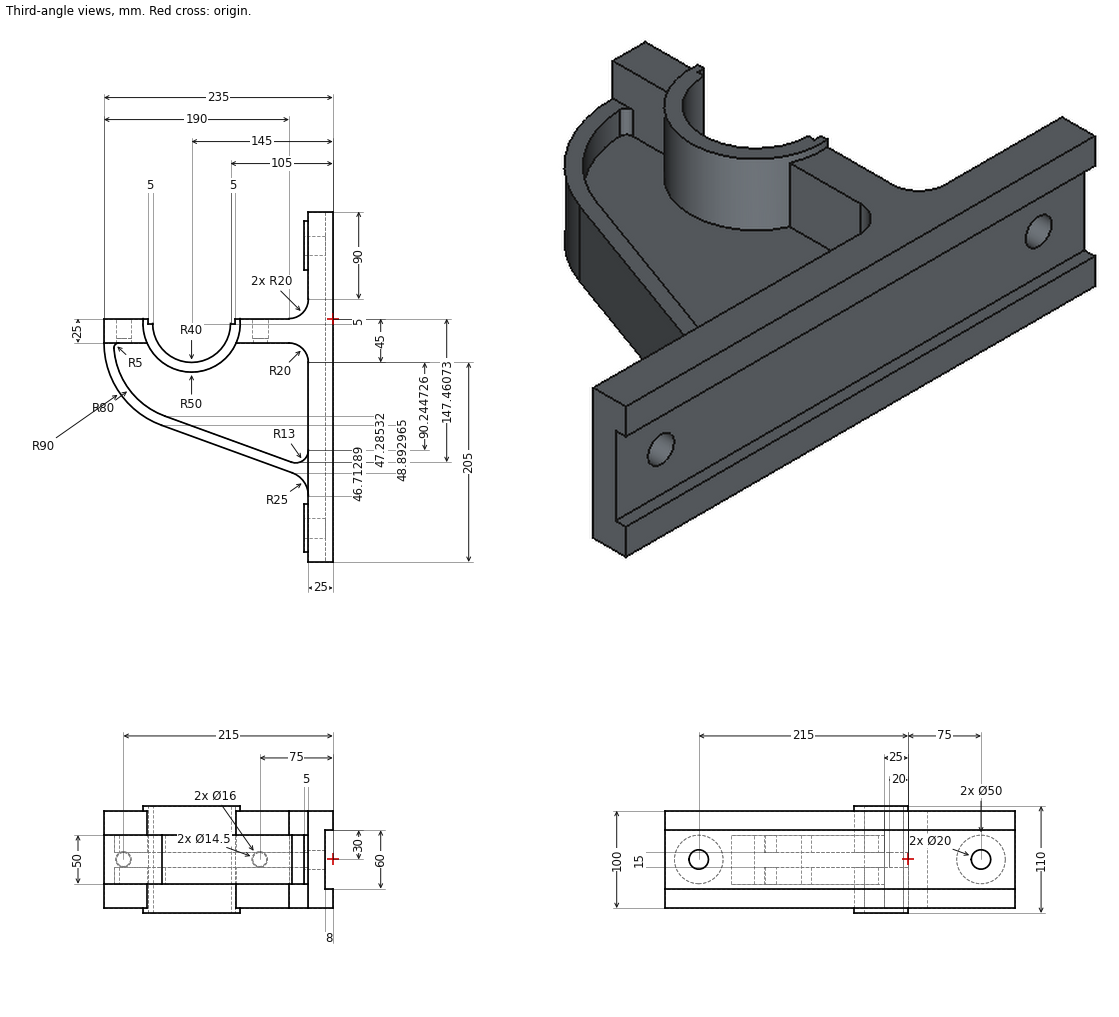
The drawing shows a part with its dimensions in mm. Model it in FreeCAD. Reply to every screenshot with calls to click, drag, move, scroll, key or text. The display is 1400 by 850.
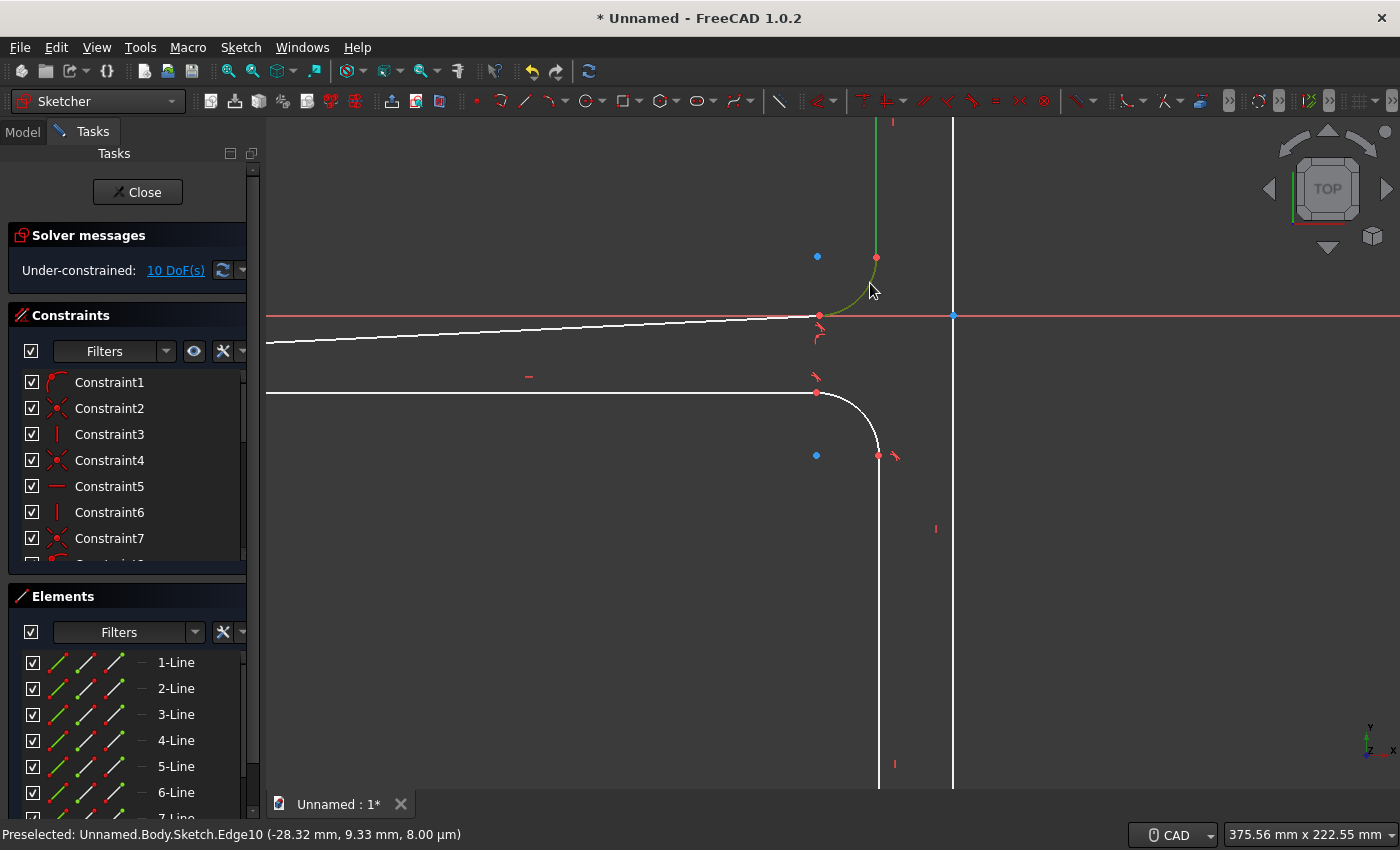
click(972, 102)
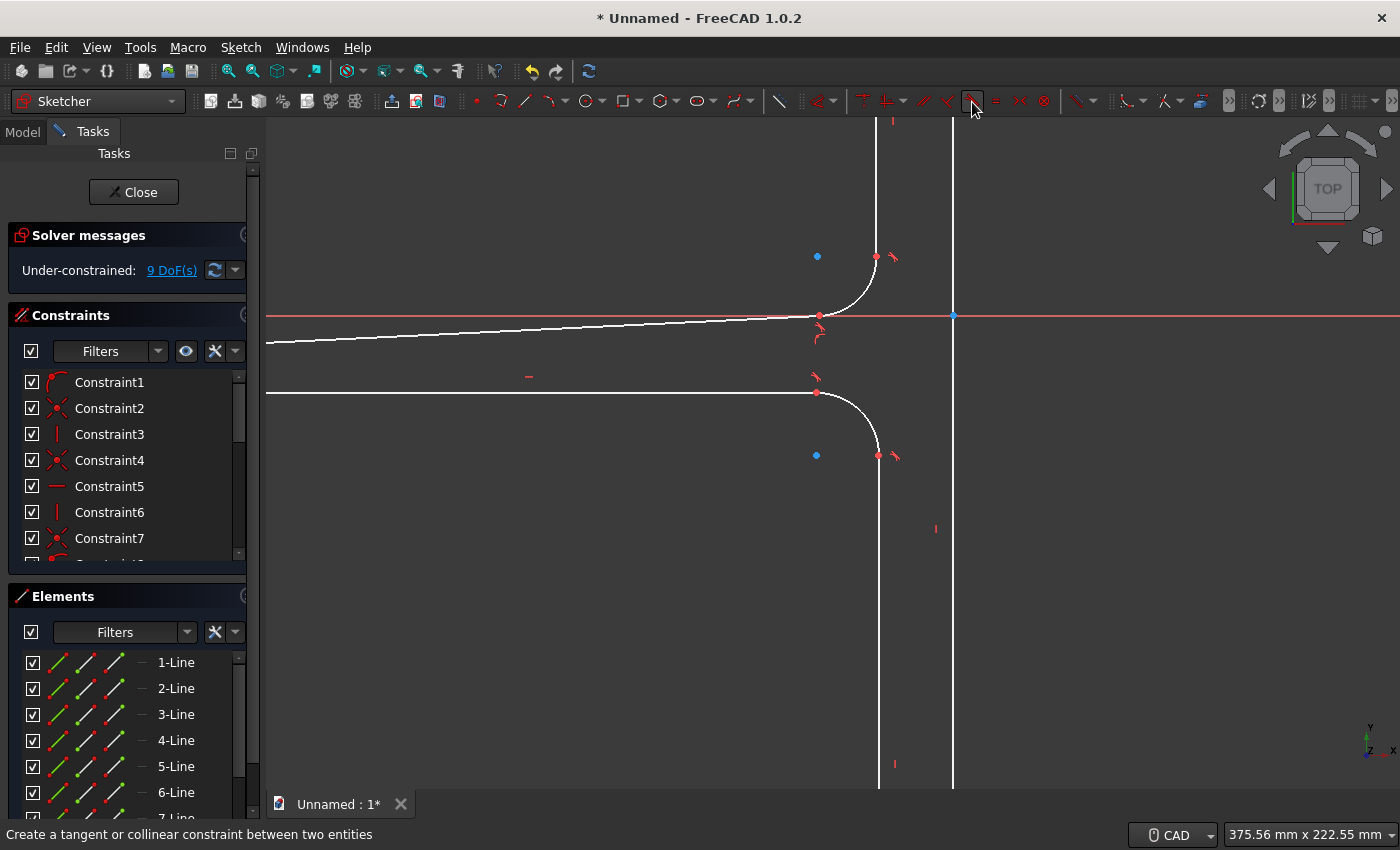
click(416, 336)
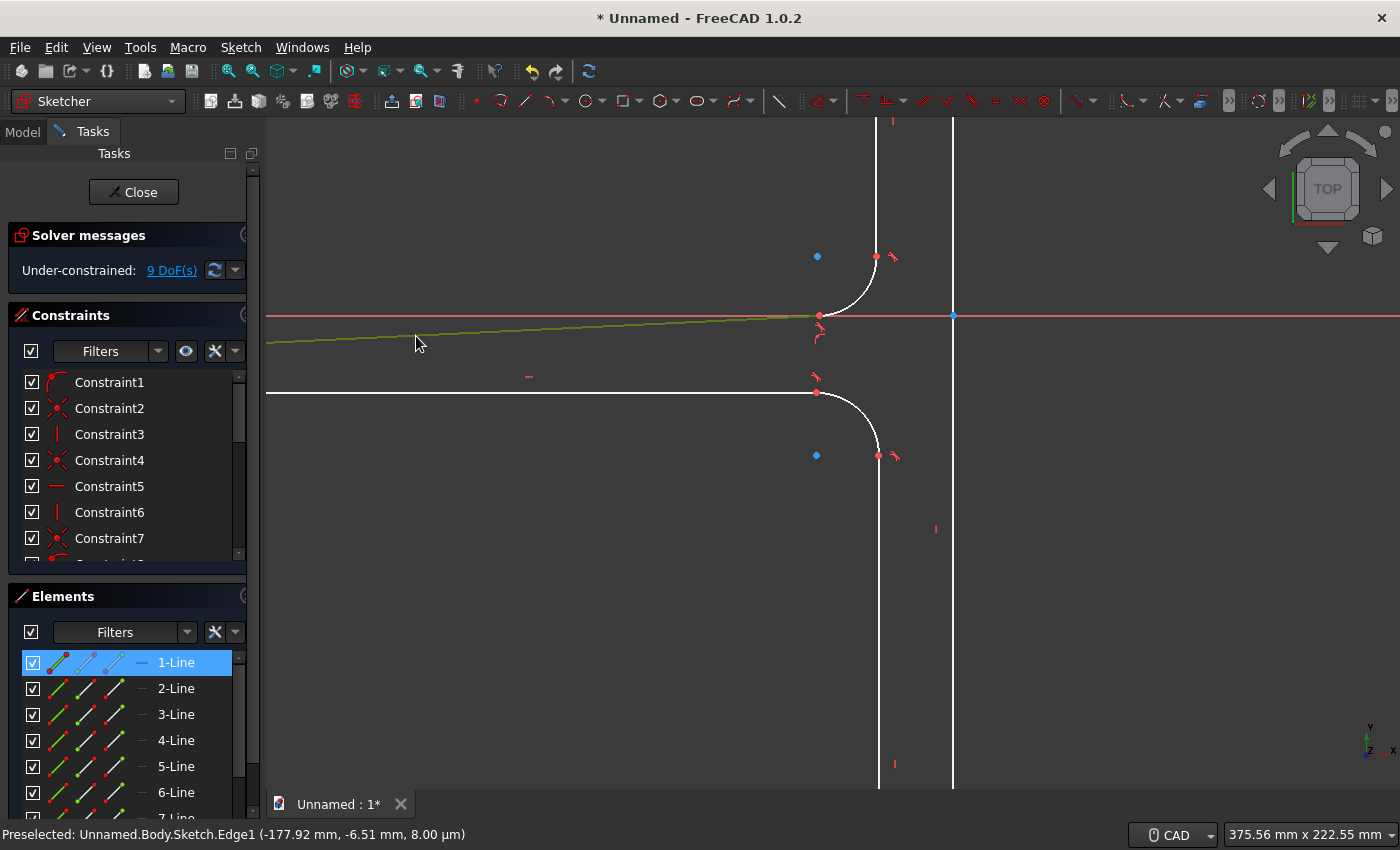
key(h)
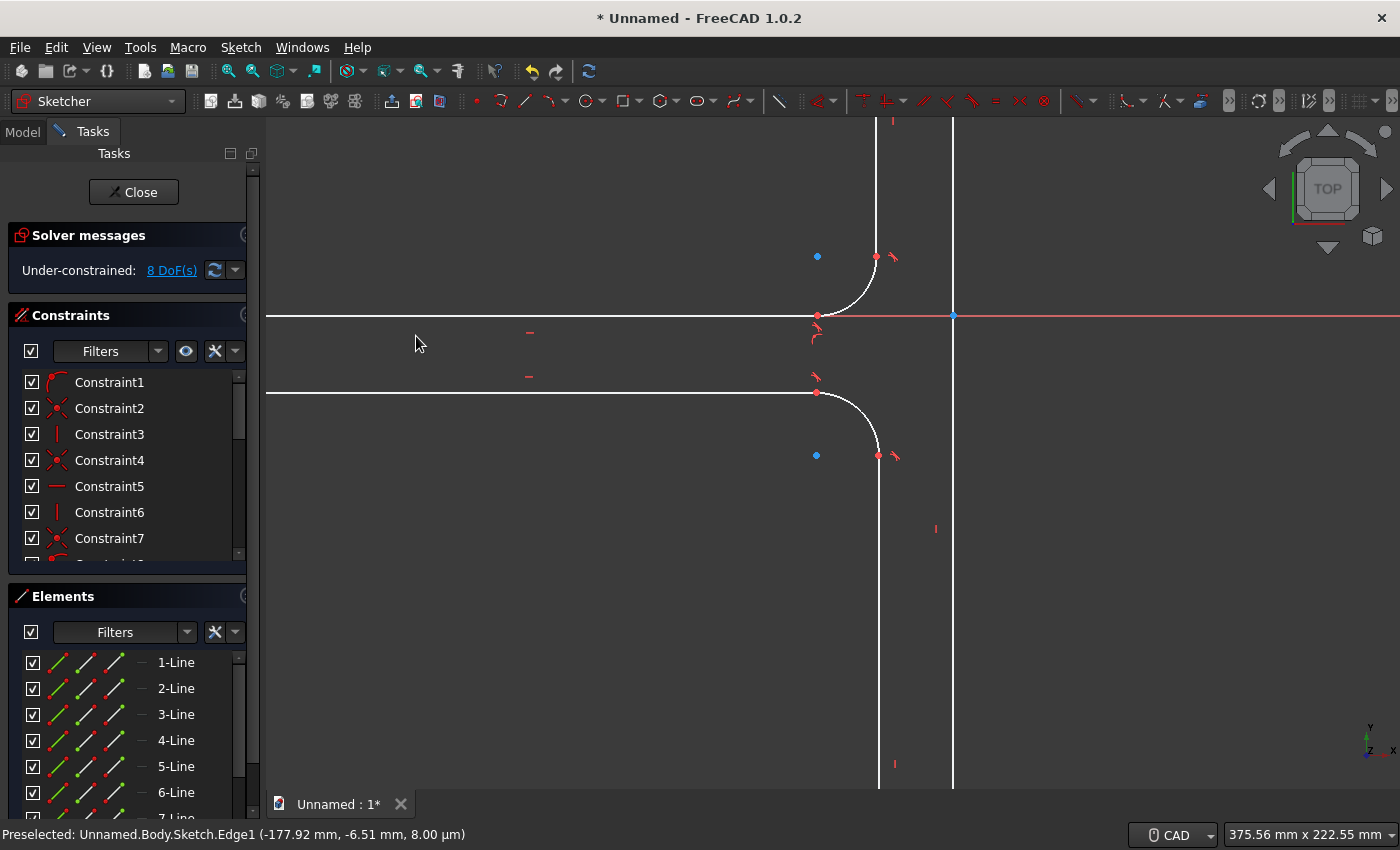
click(872, 427)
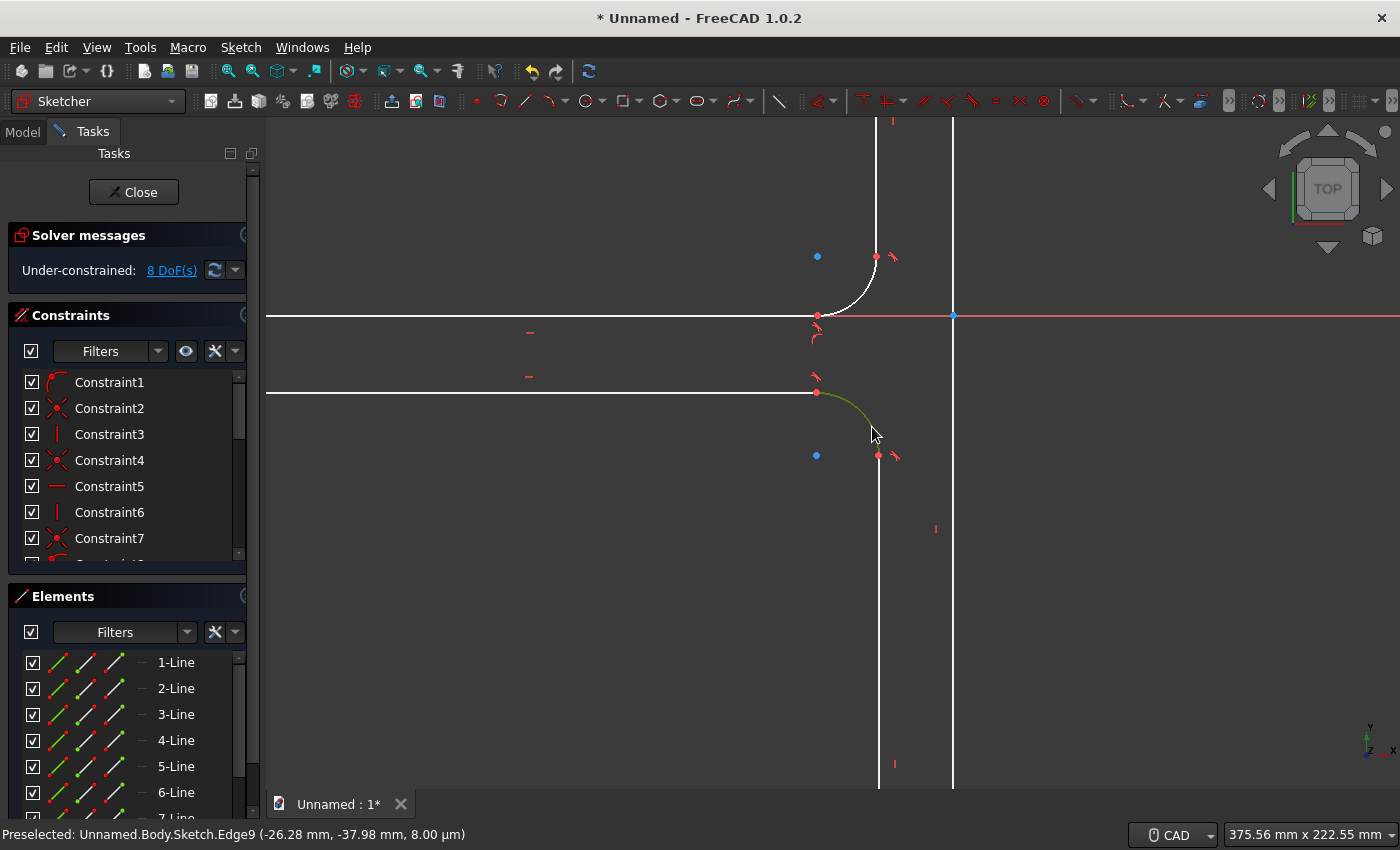
click(870, 284)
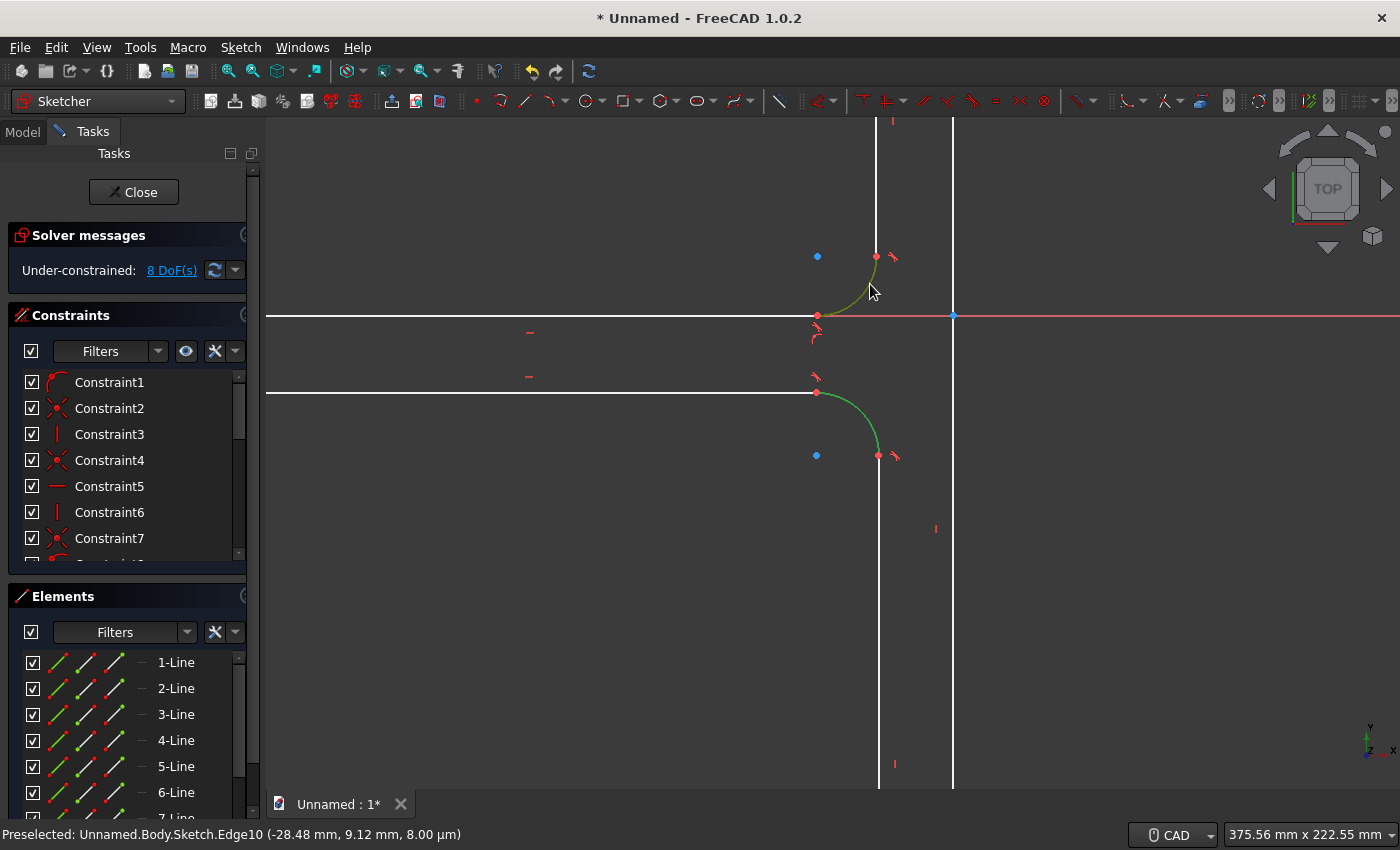
click(996, 102)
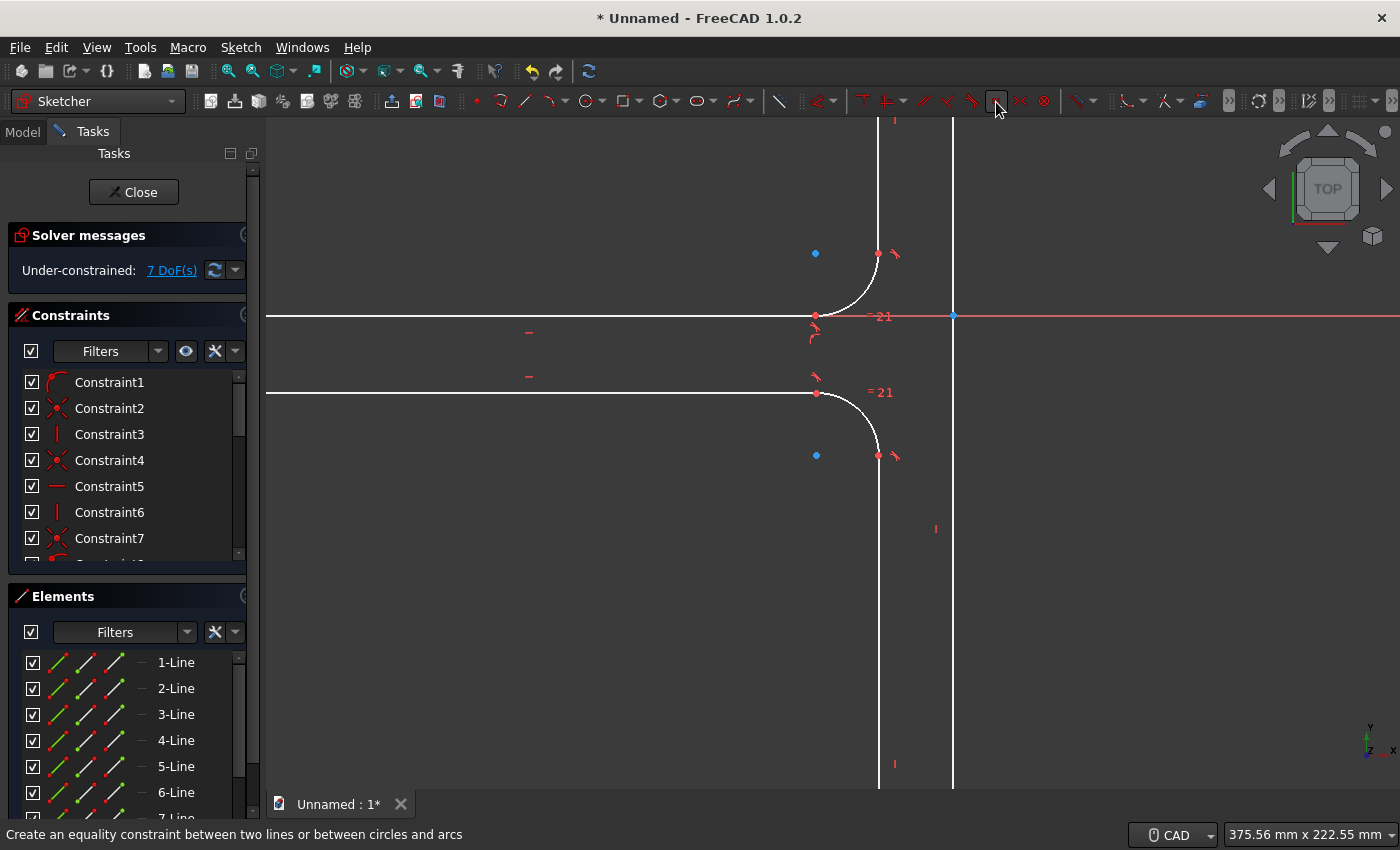
click(818, 102)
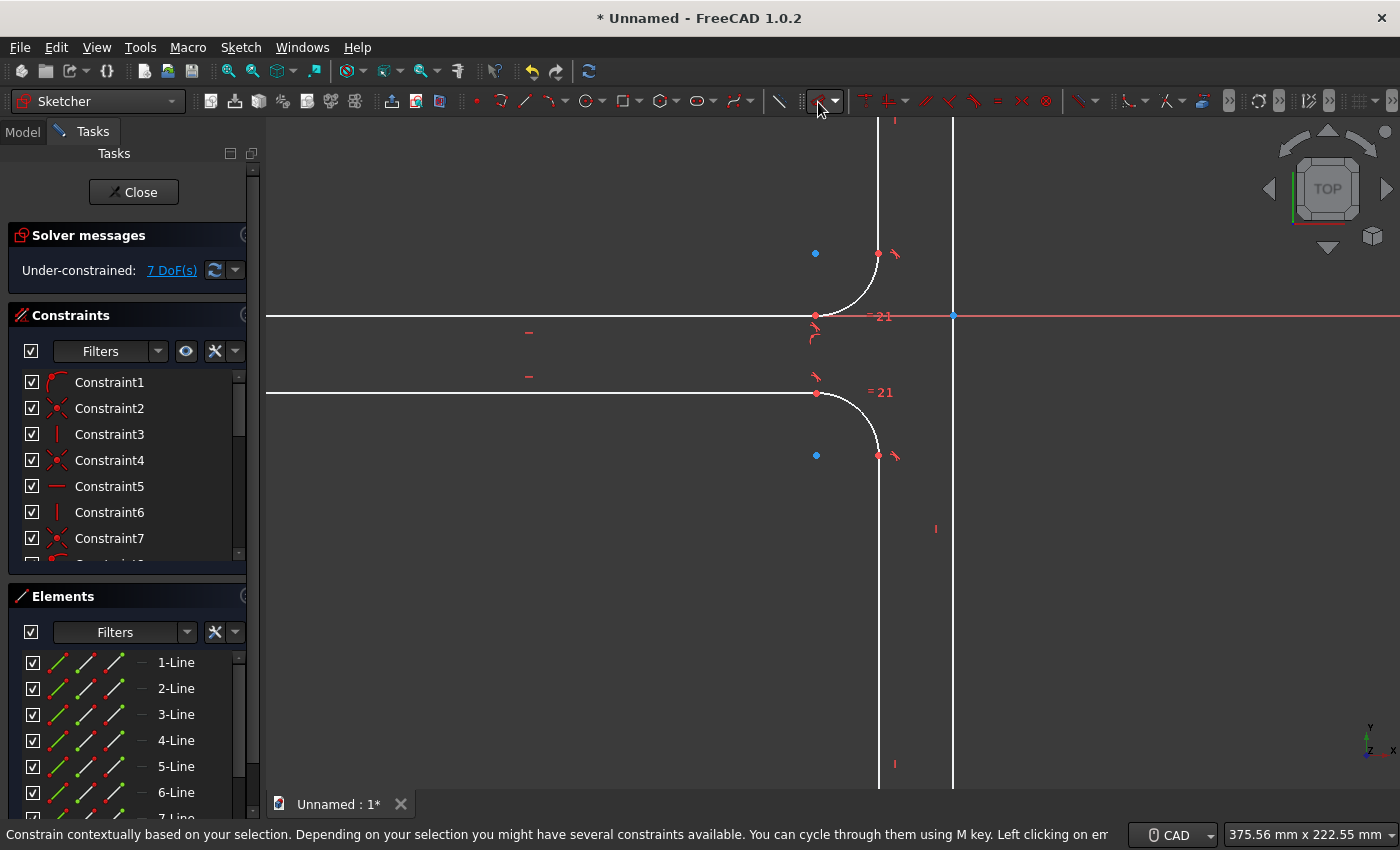
click(872, 427)
click(900, 412)